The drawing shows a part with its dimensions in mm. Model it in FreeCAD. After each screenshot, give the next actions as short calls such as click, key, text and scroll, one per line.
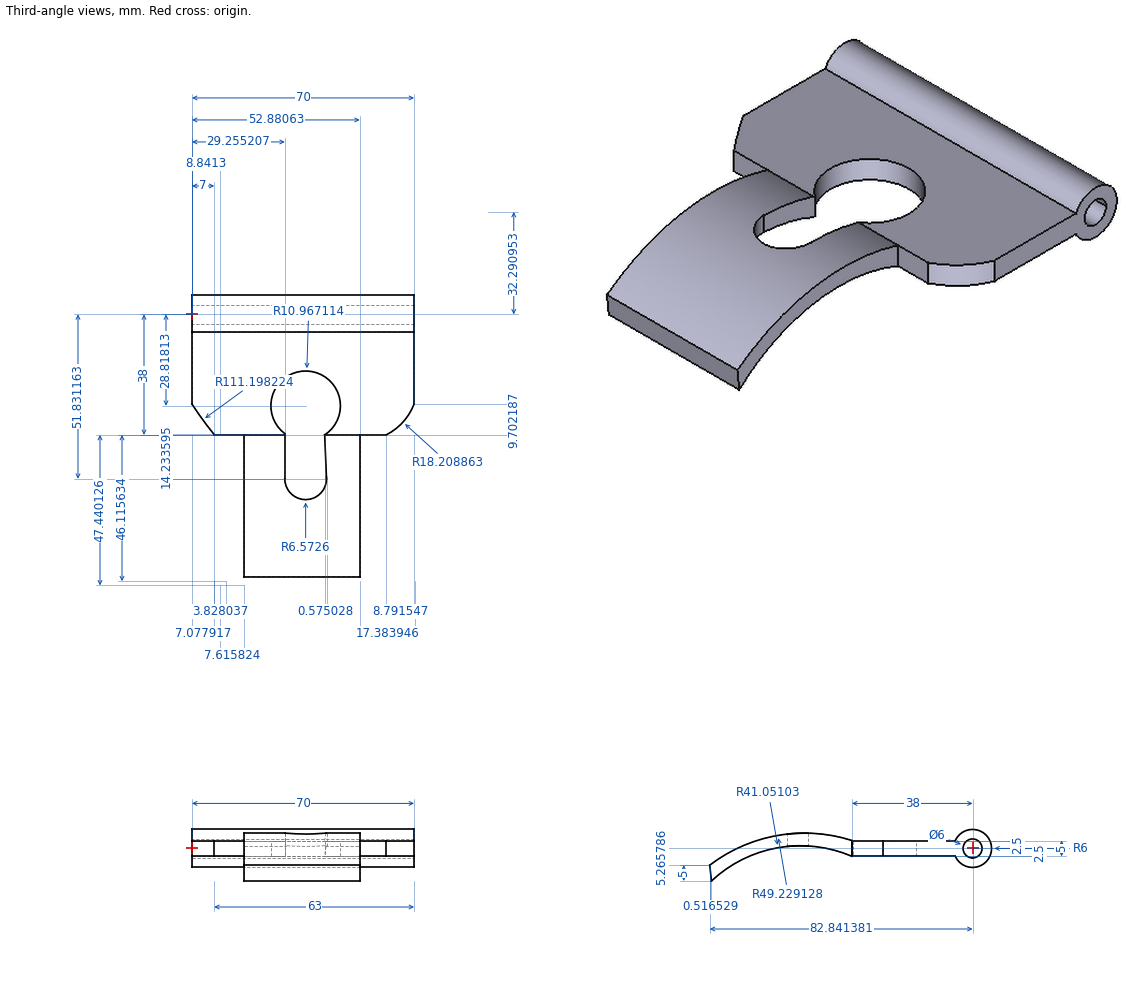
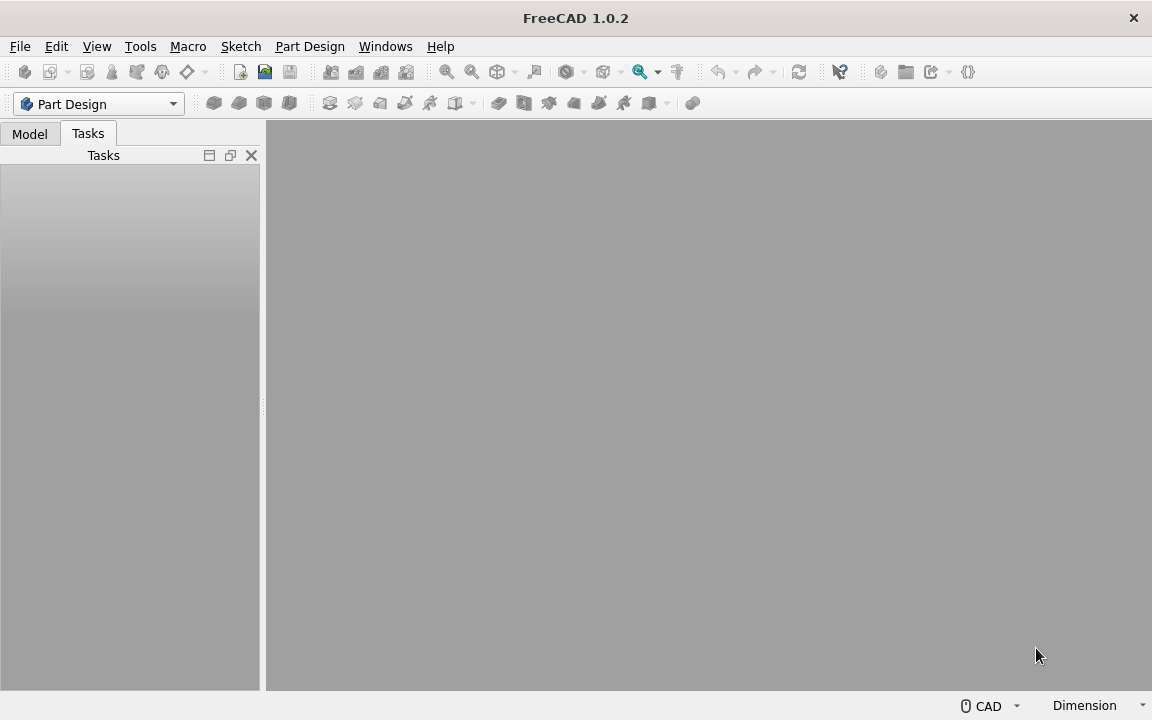
click(240, 72)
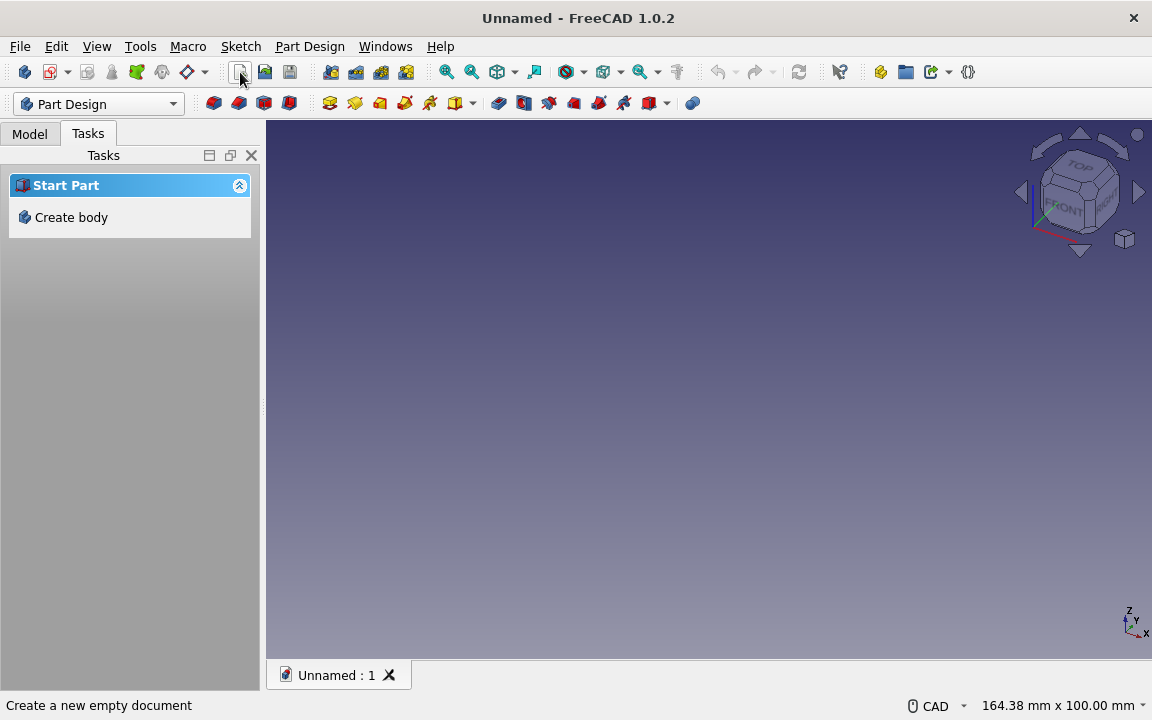
click(50, 72)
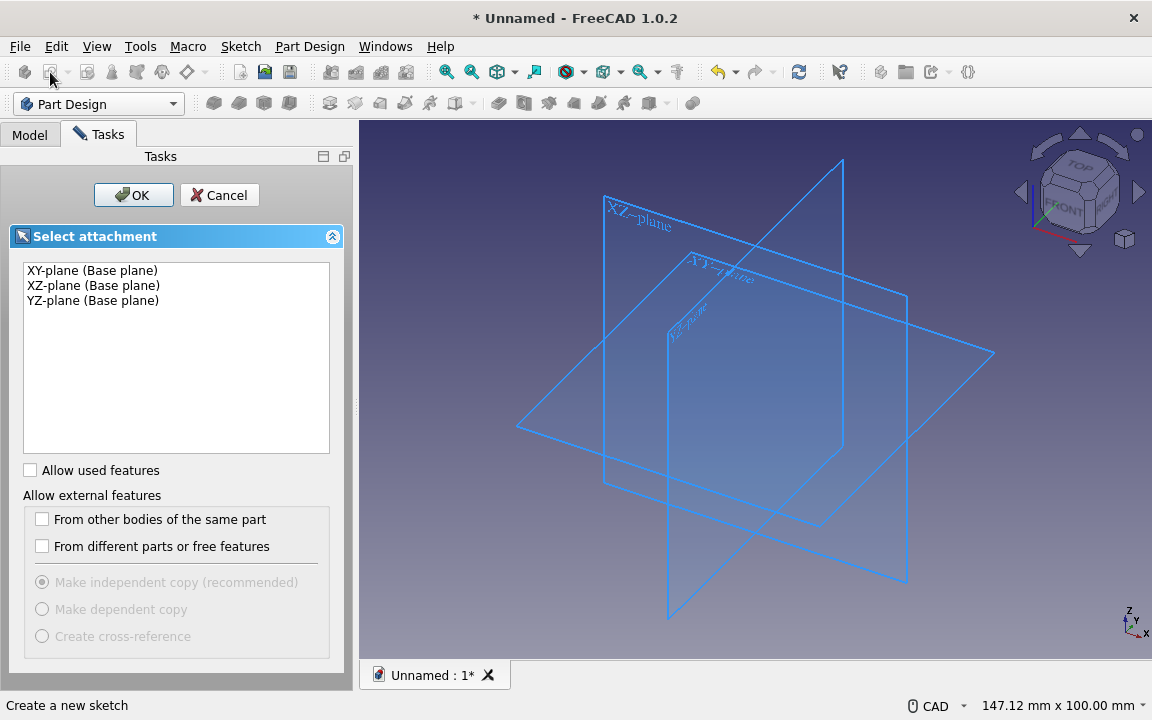
click(84, 300)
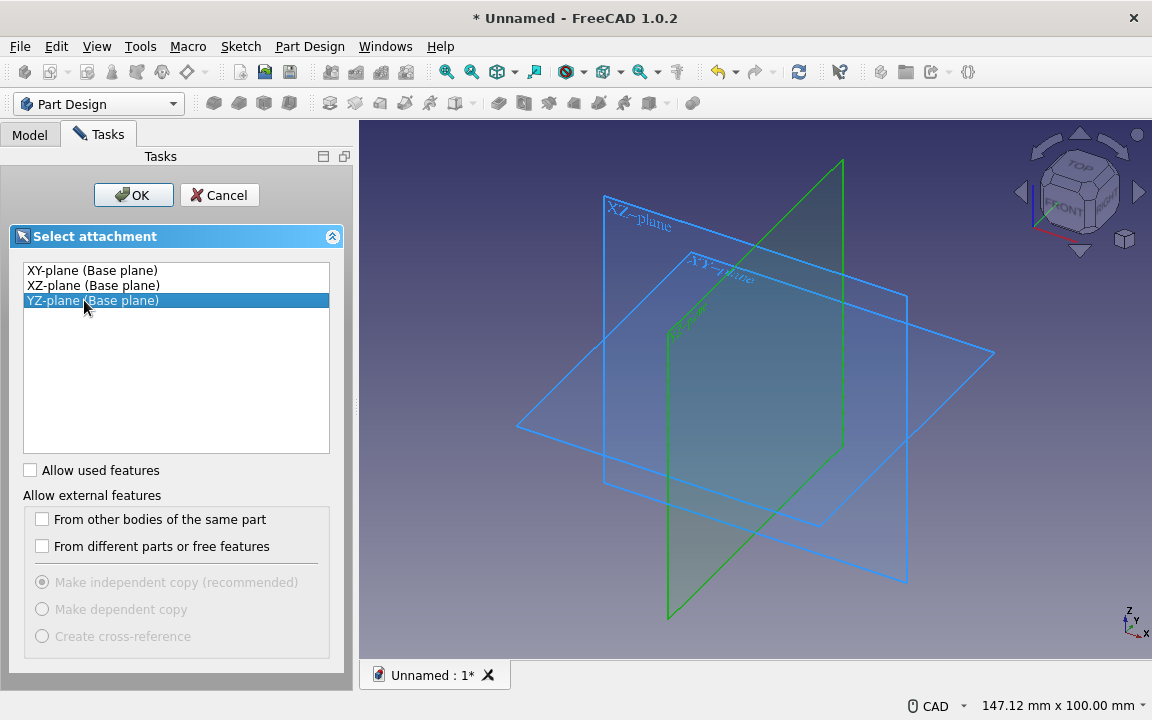
click(134, 195)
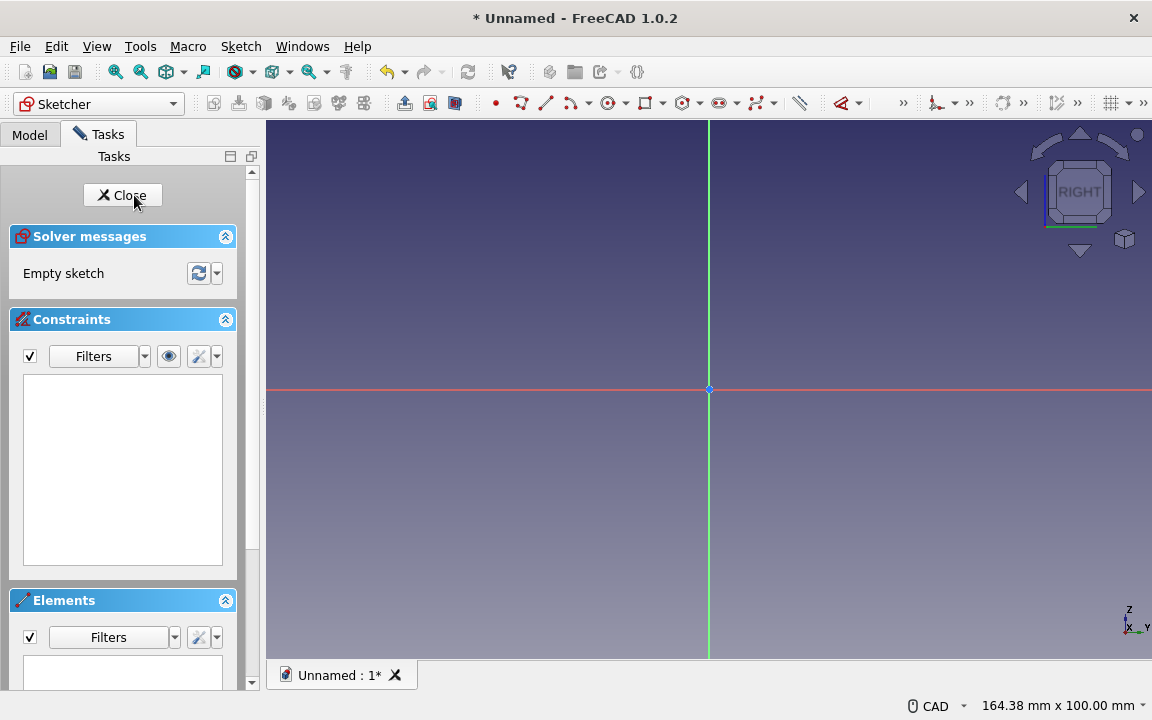
scroll(608, 390, up, 4)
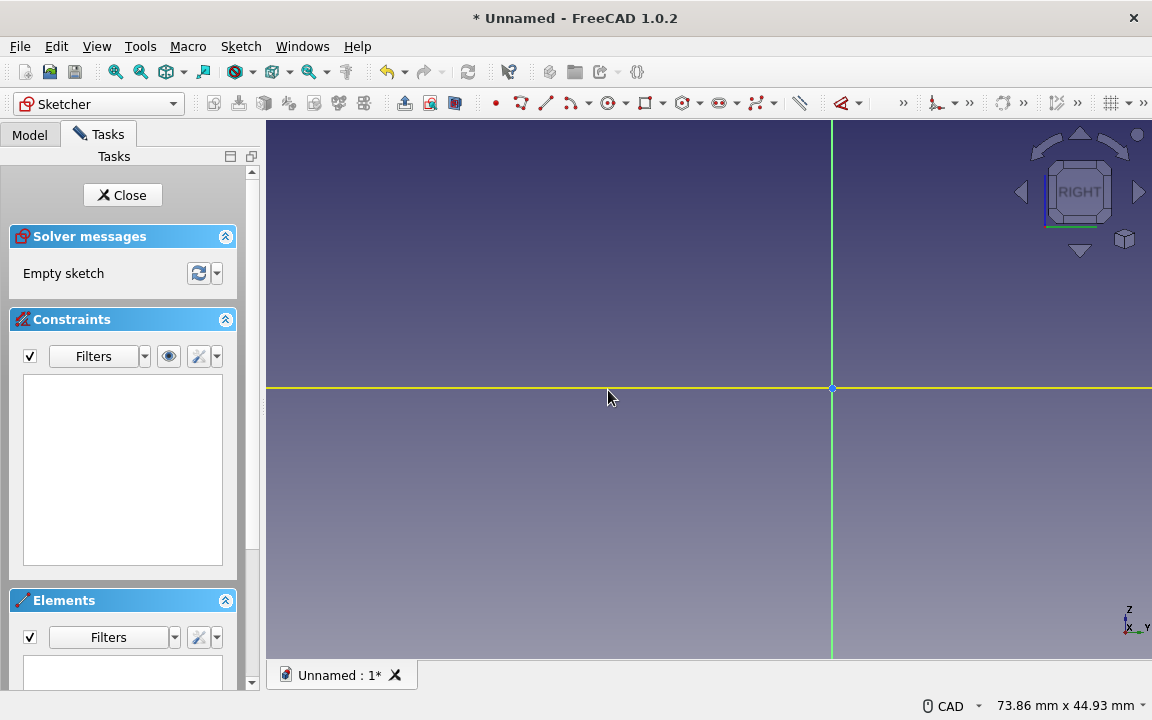
click(521, 104)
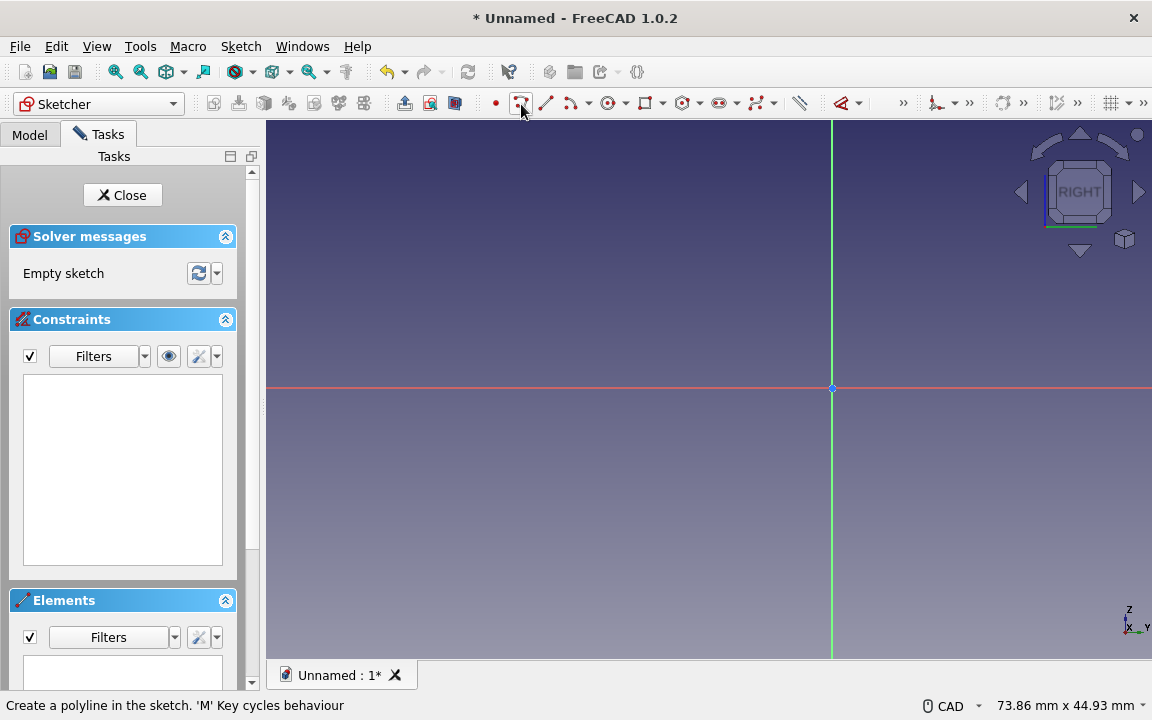
click(767, 358)
click(376, 358)
click(376, 418)
click(767, 418)
right_click(767, 418)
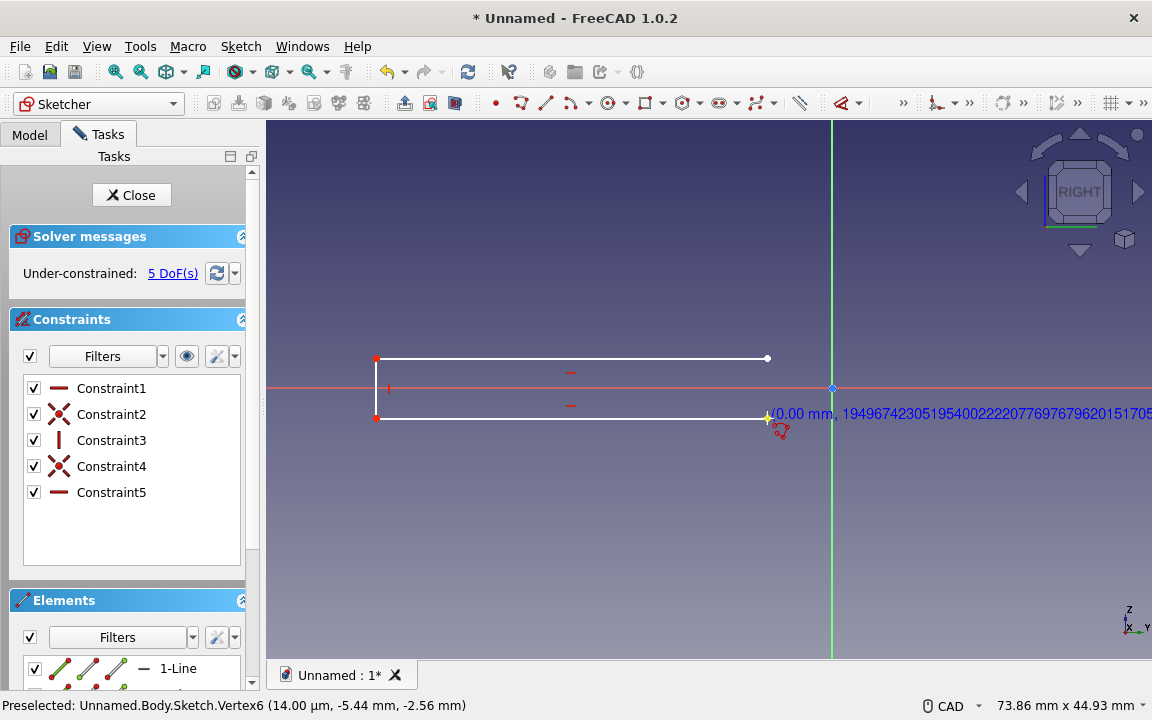
click(588, 104)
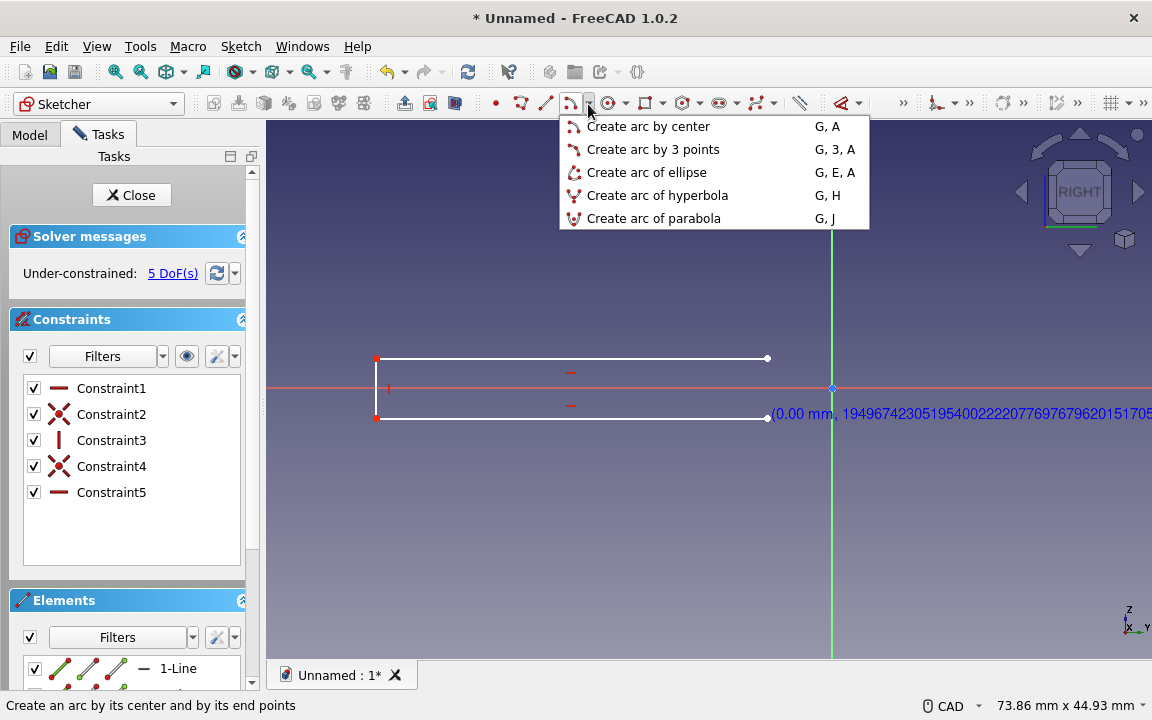
click(714, 150)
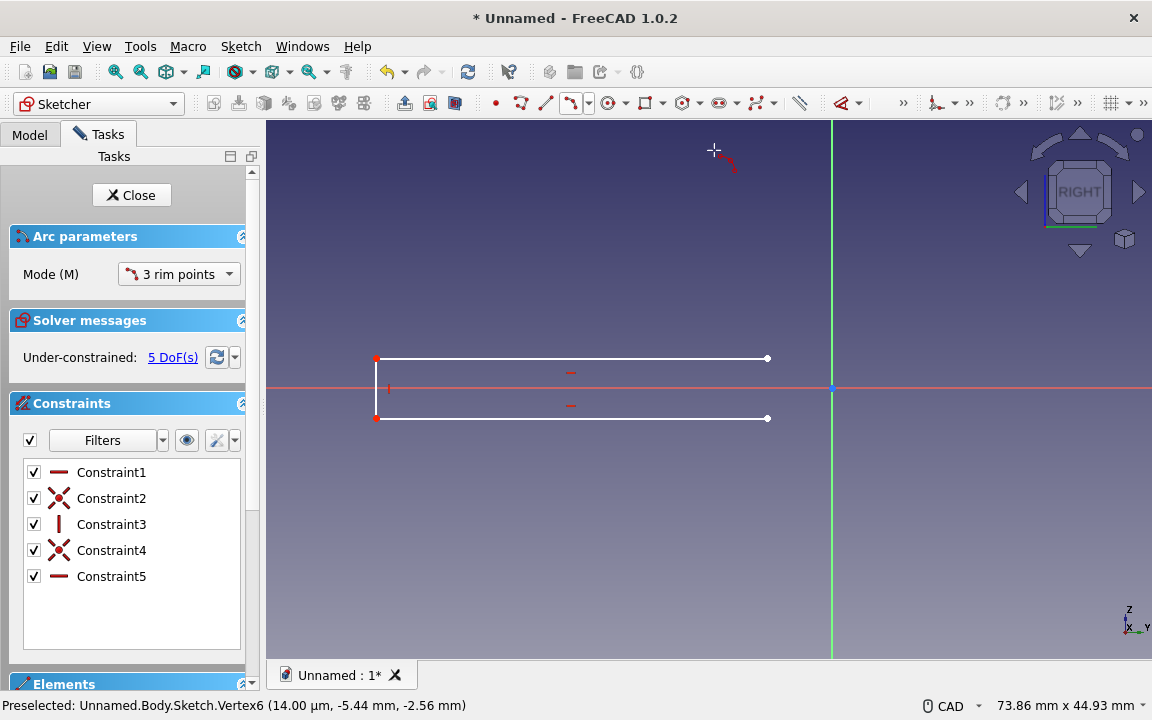
click(767, 419)
click(767, 359)
click(894, 425)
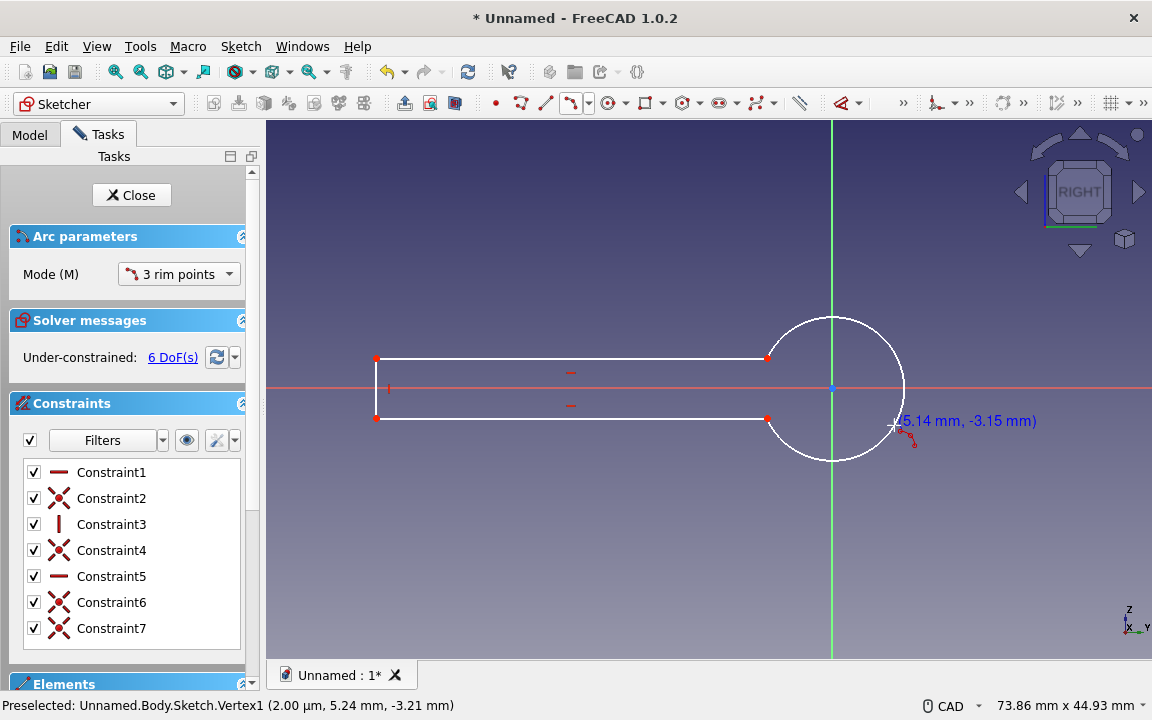
click(608, 104)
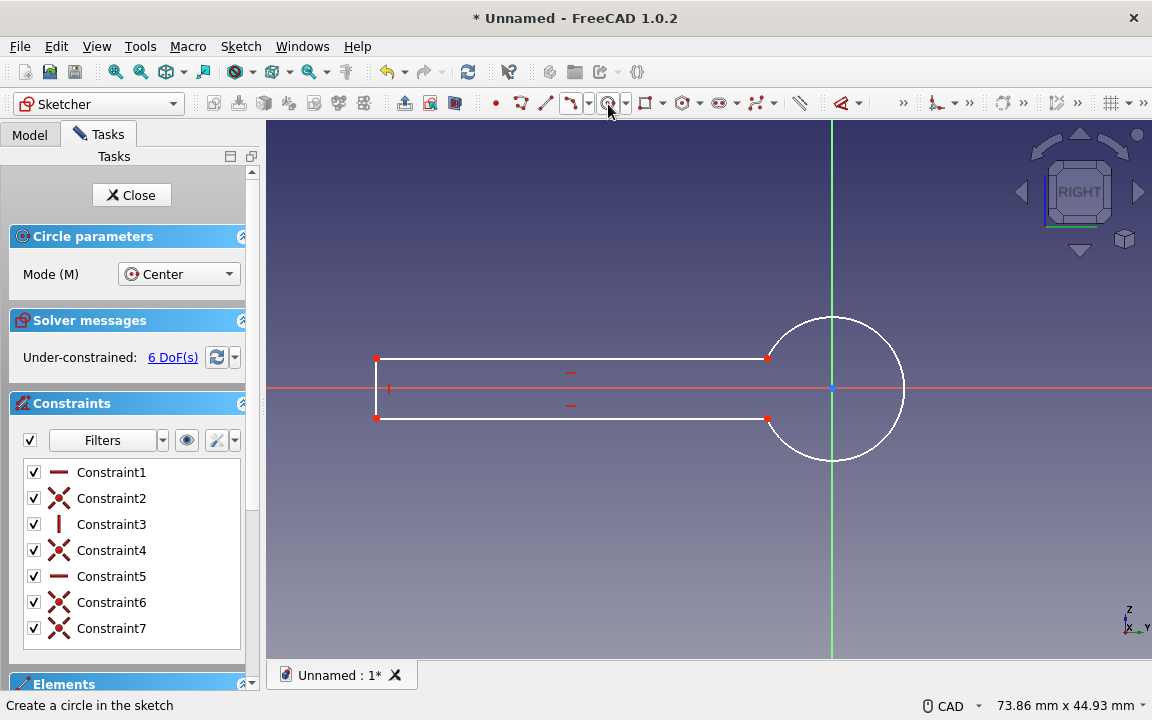
click(832, 388)
move(858, 363)